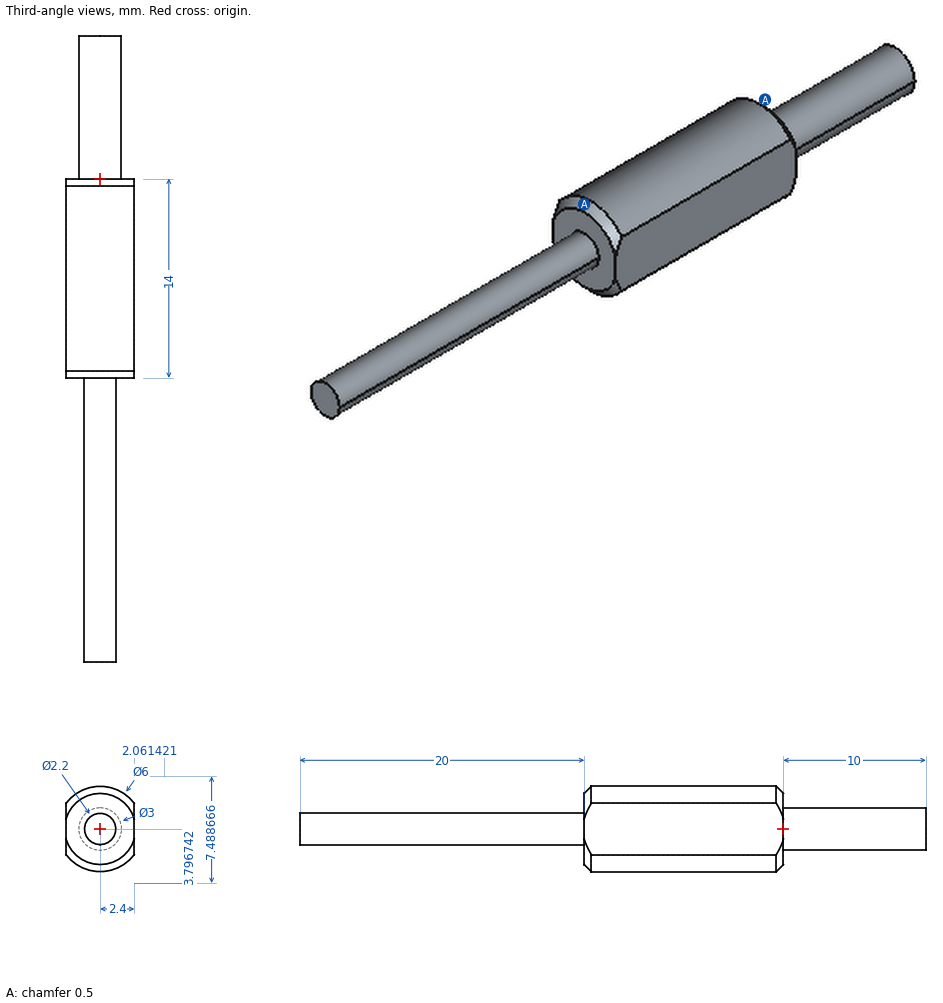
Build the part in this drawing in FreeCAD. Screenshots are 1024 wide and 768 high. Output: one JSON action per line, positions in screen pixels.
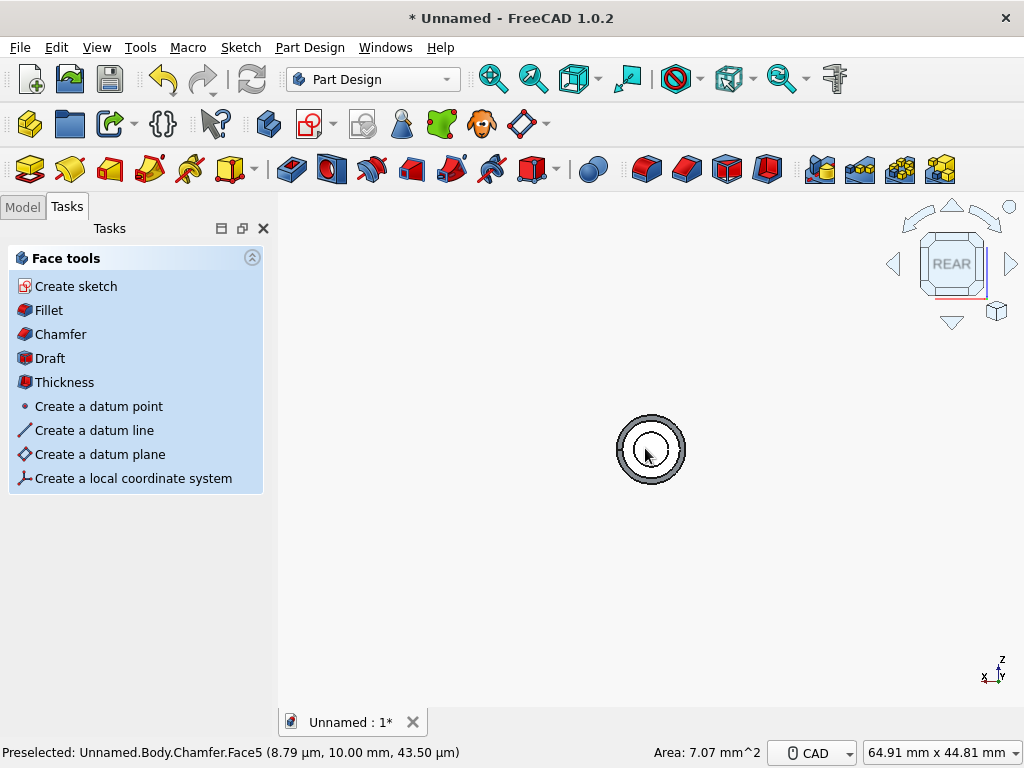
{"action": "left_click", "coordinate": [310, 124]}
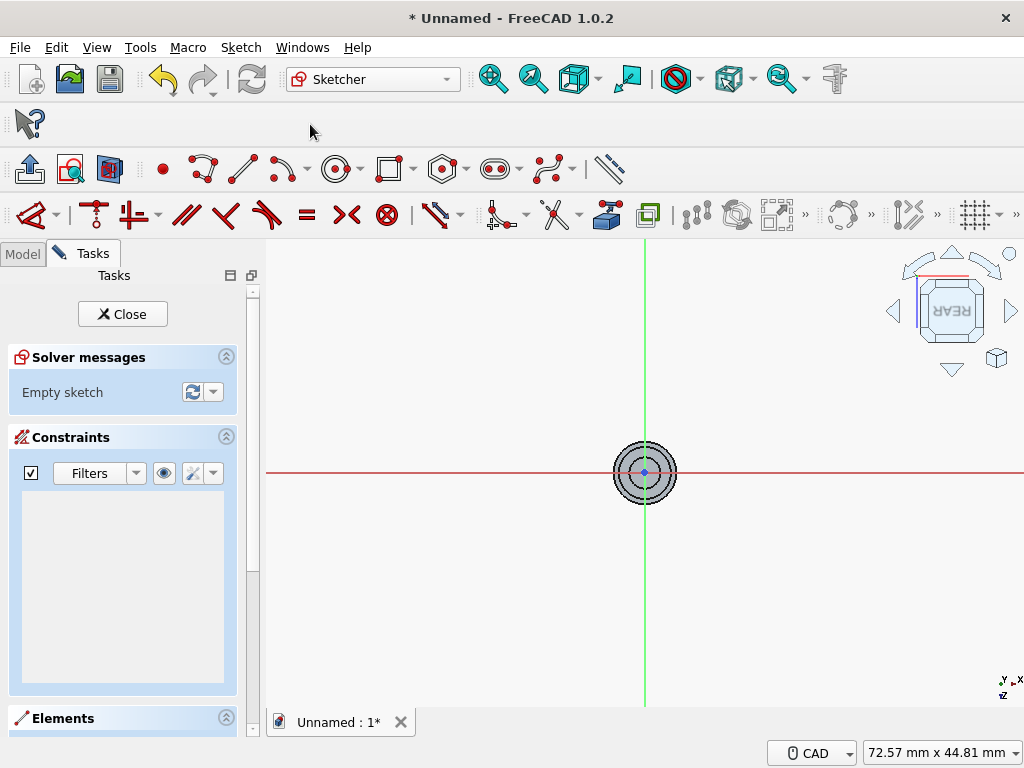
{"action": "scroll", "coordinate": [698, 472], "scroll_direction": "up", "scroll_amount": 7}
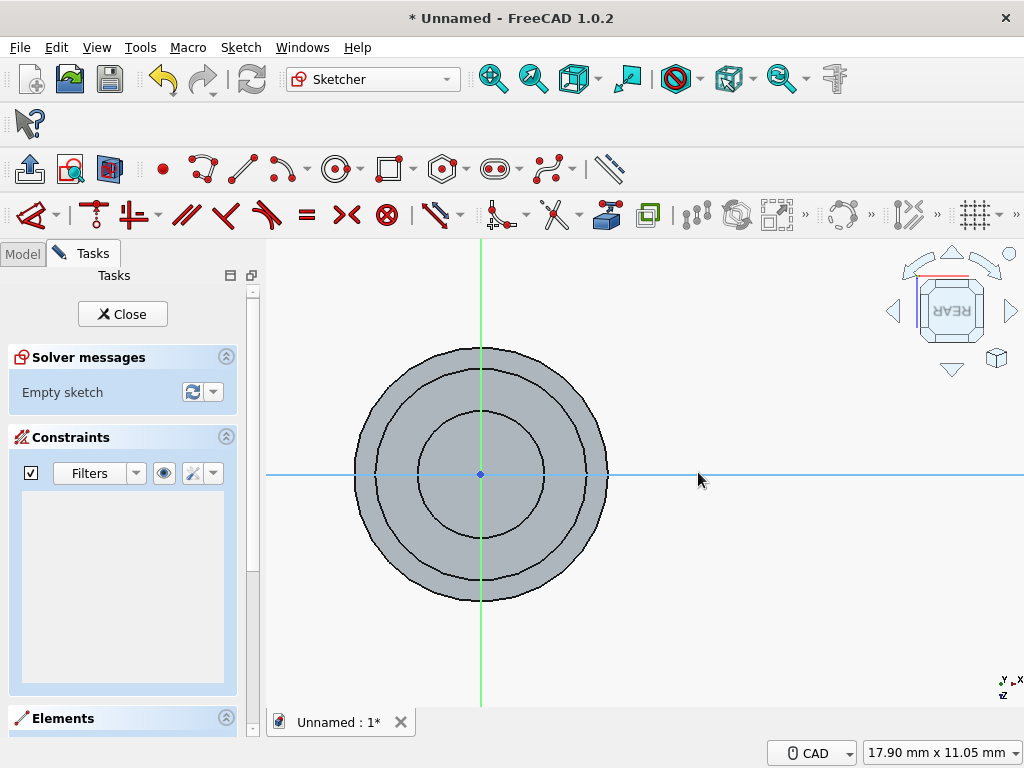
{"action": "key", "text": "g r"}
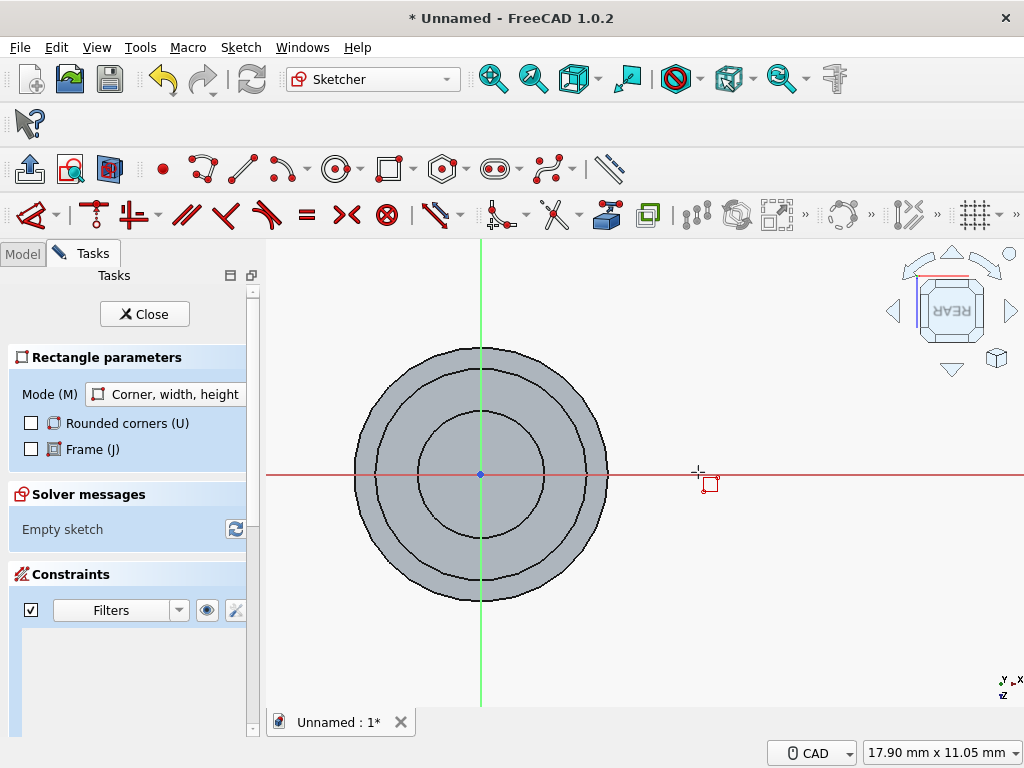
{"action": "left_click", "coordinate": [583, 314]}
{"action": "left_click", "coordinate": [670, 631]}
{"action": "key", "text": "Escape"}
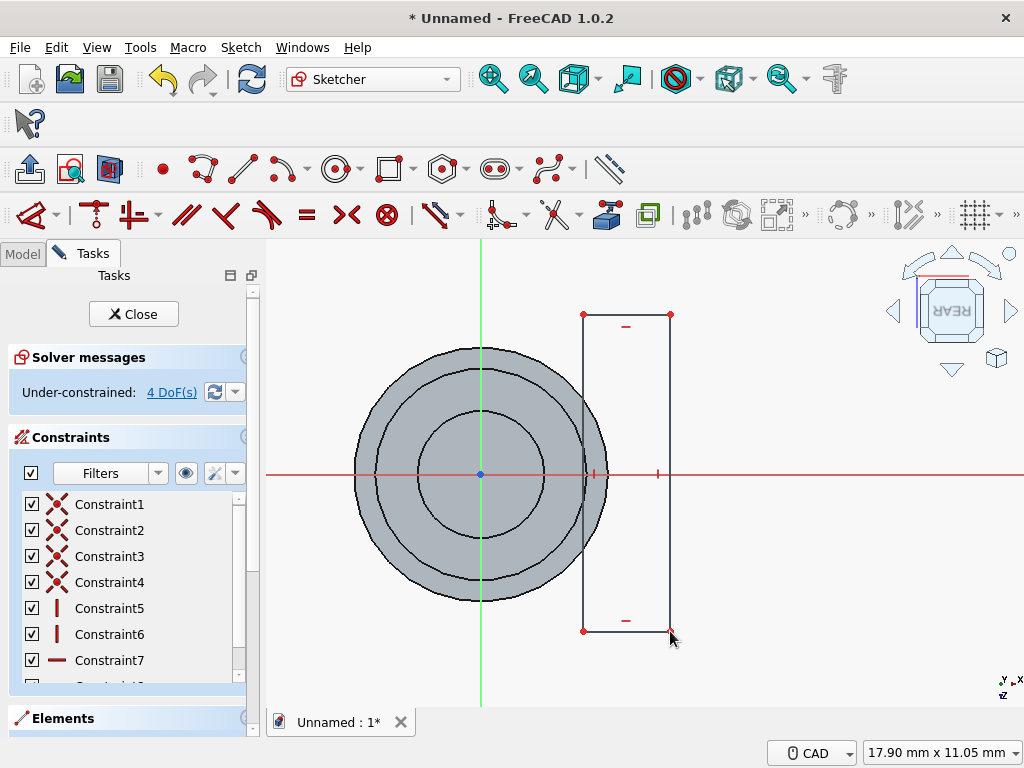
{"action": "left_click", "coordinate": [32, 216]}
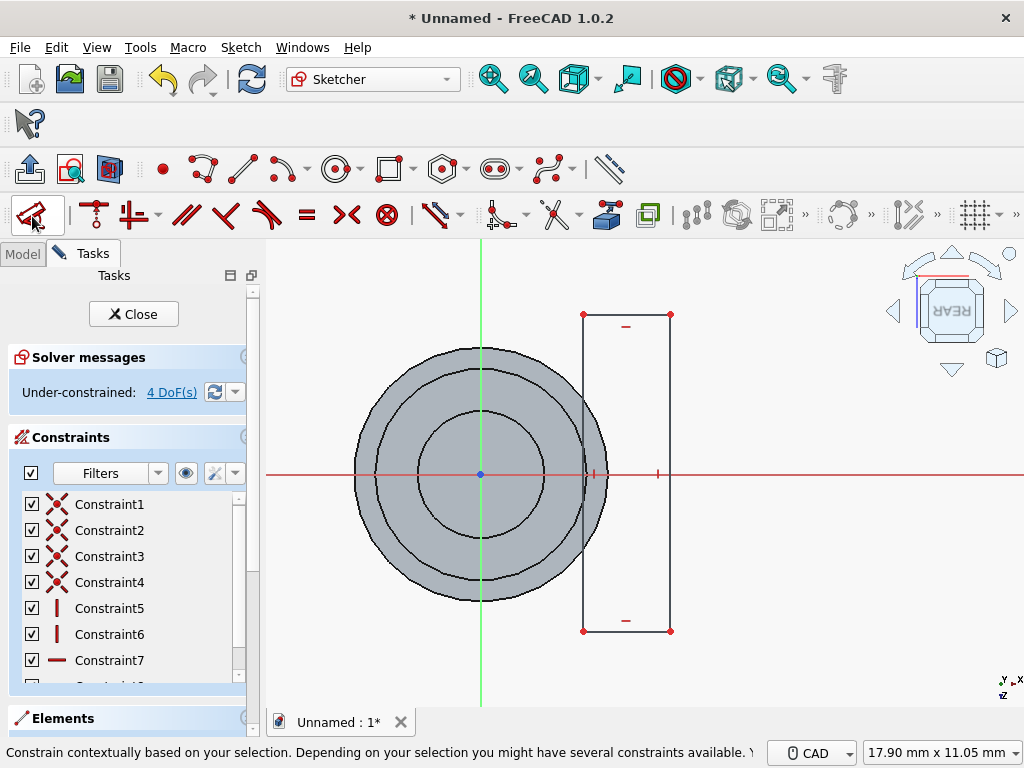
{"action": "left_click", "coordinate": [583, 315]}
{"action": "left_click", "coordinate": [532, 281]}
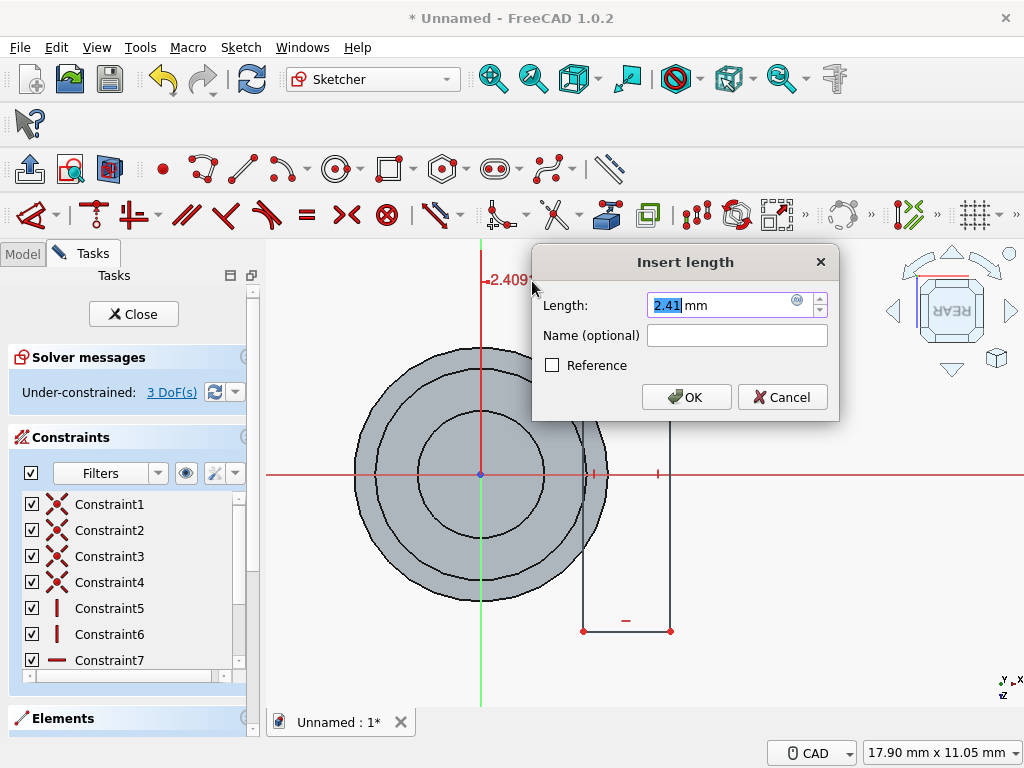
{"action": "type", "text": "2.4"}
{"action": "key", "text": "Return"}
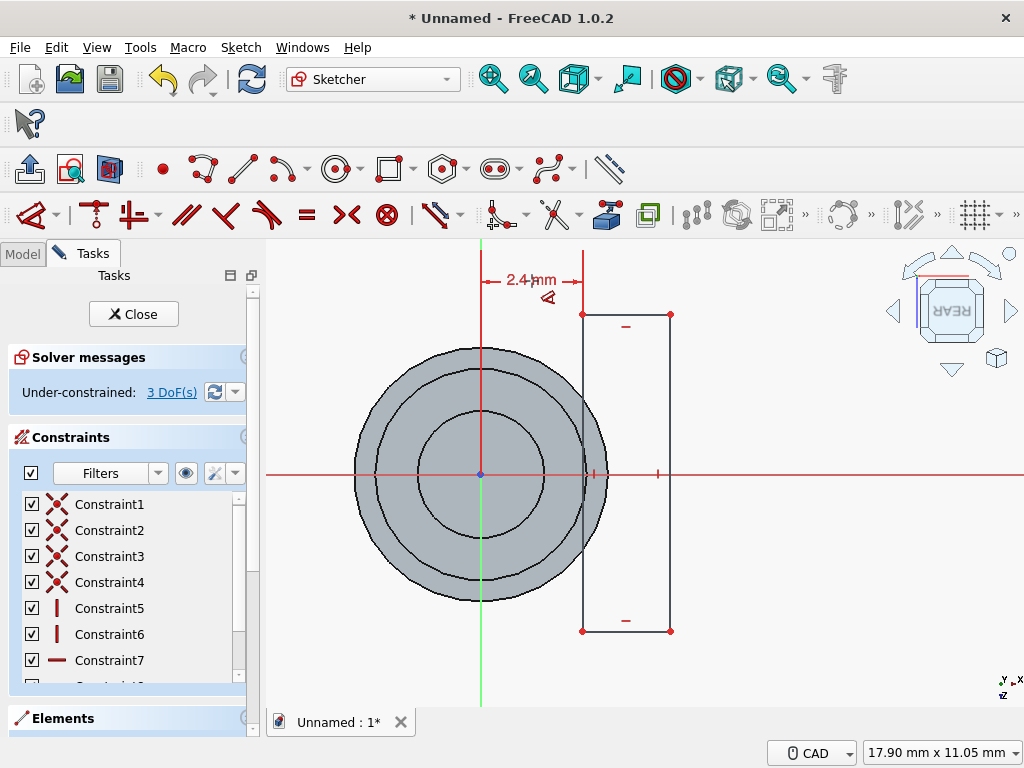
{"action": "left_click", "coordinate": [583, 410]}
{"action": "left_click", "coordinate": [617, 401]}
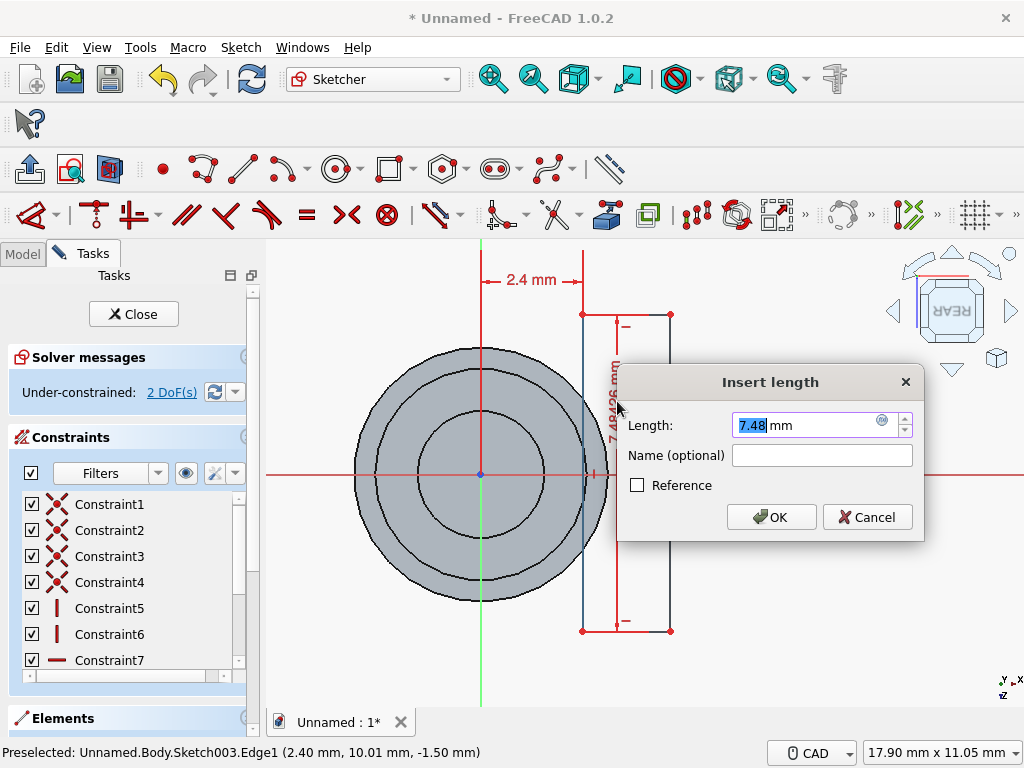
{"action": "type", "text": "7.488666"}
{"action": "key", "text": "Return"}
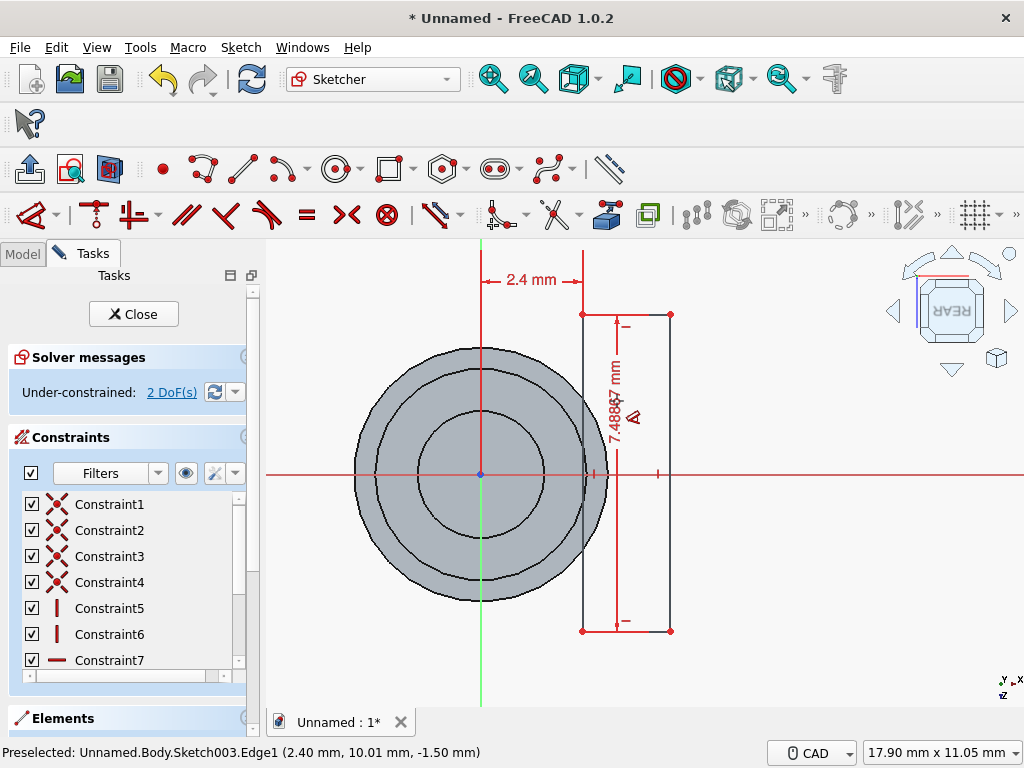
{"action": "left_click", "coordinate": [609, 632]}
{"action": "left_click", "coordinate": [626, 666]}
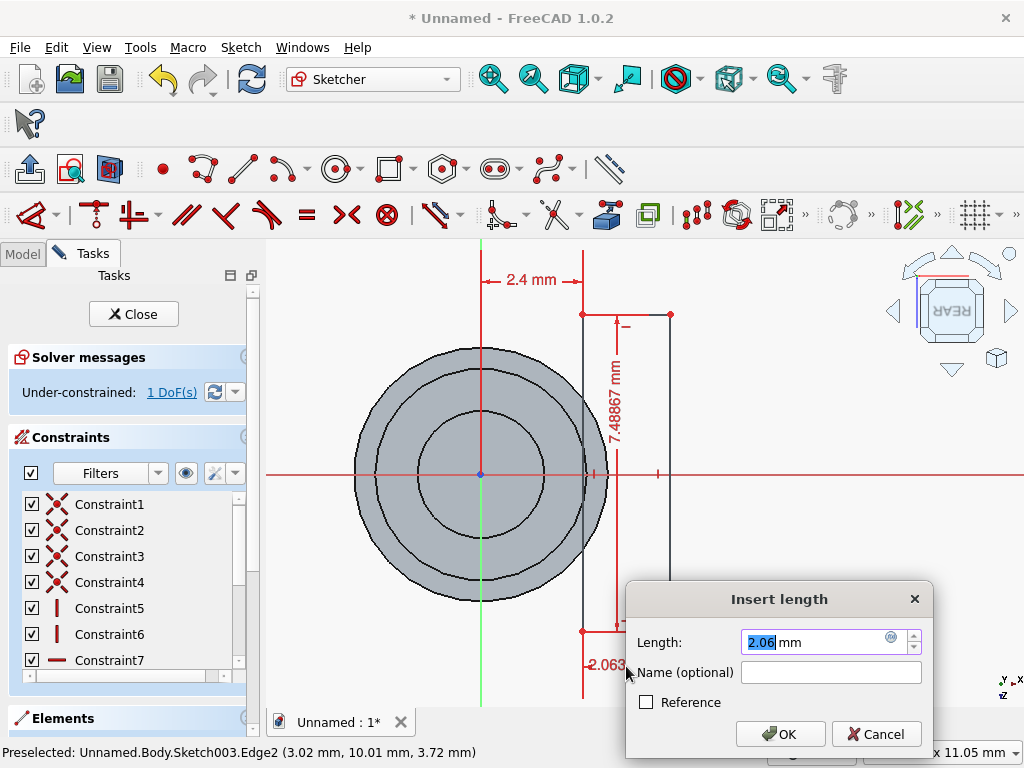
{"action": "type", "text": "2.061421"}
{"action": "key", "text": "Return"}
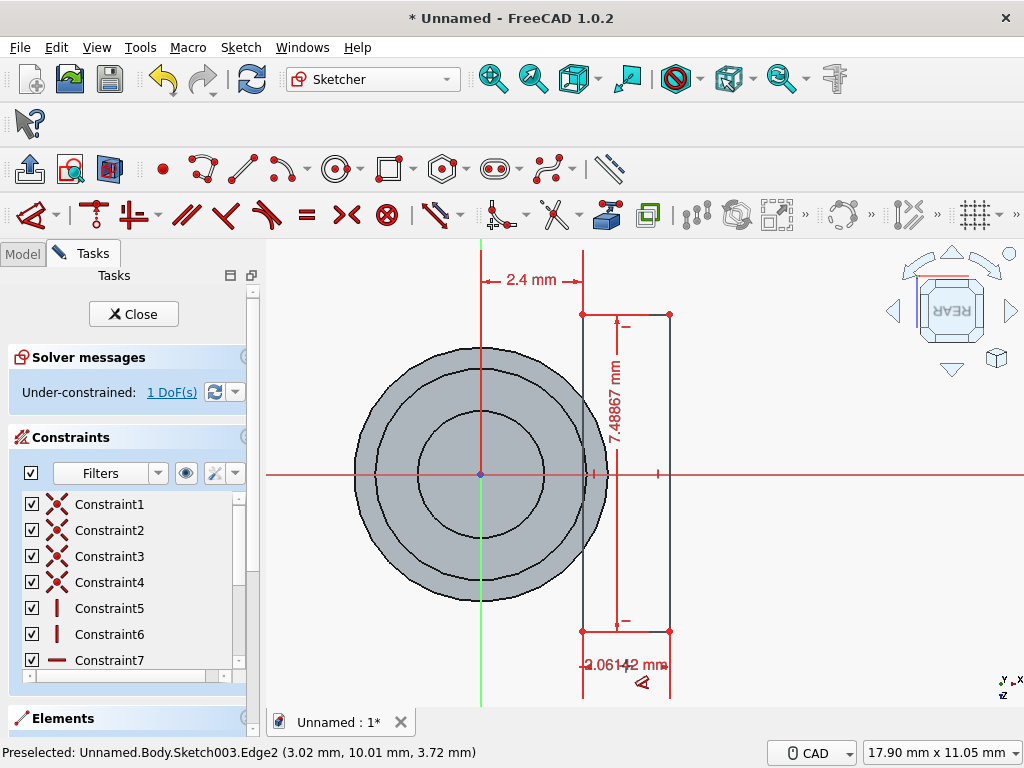
{"action": "left_click", "coordinate": [583, 315]}
{"action": "left_click", "coordinate": [447, 395]}